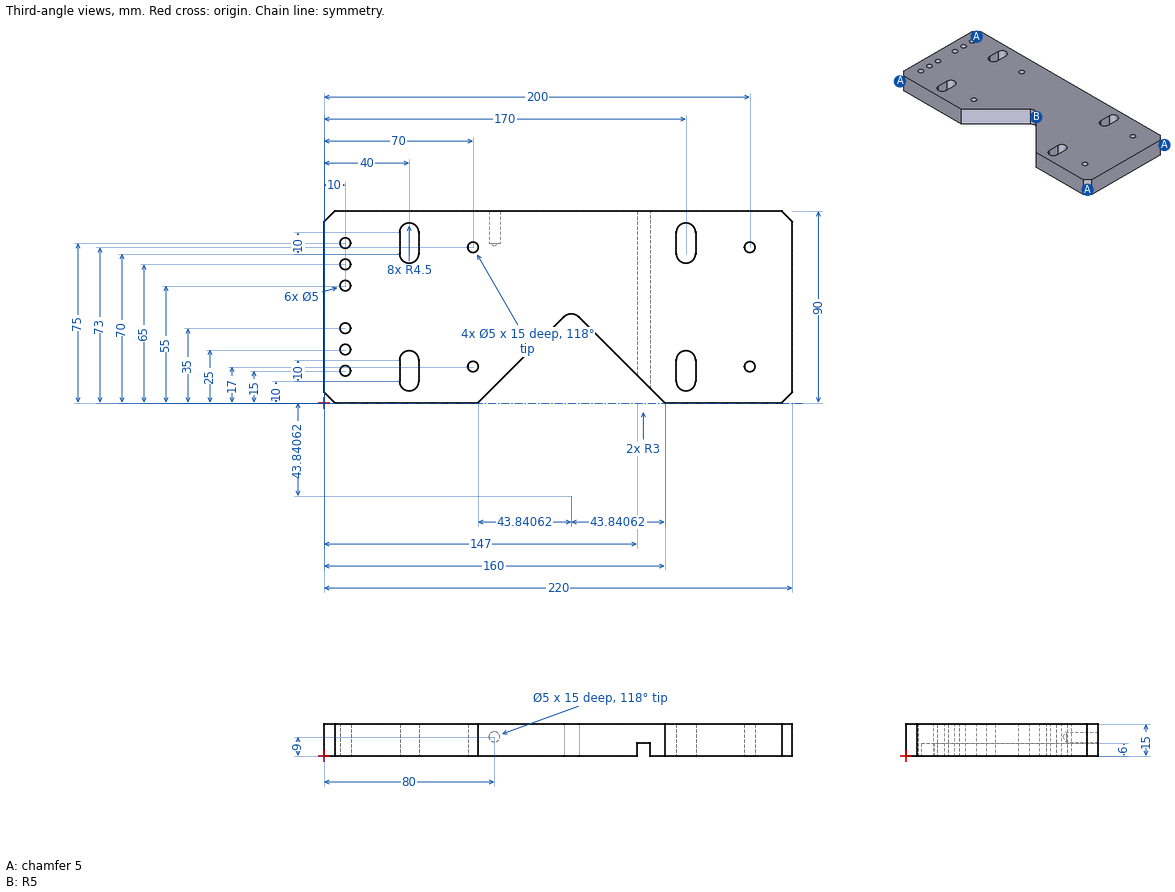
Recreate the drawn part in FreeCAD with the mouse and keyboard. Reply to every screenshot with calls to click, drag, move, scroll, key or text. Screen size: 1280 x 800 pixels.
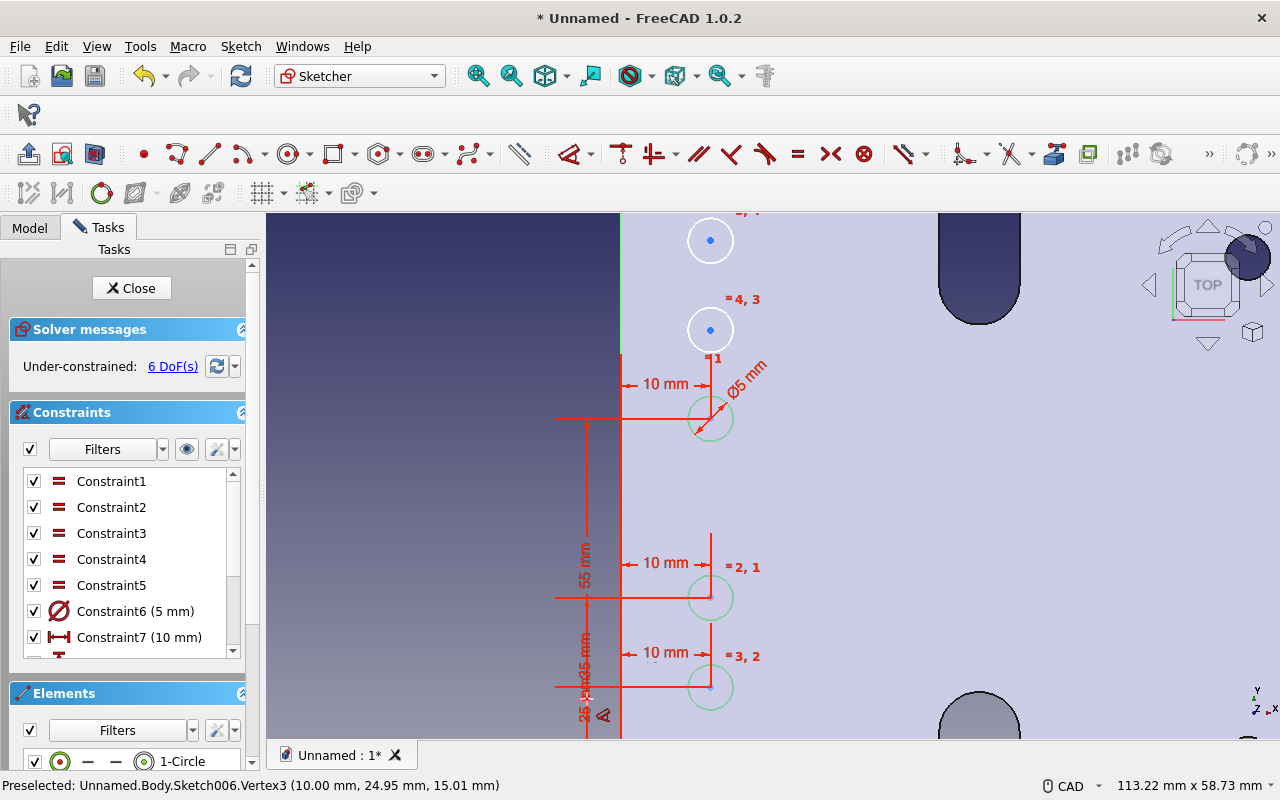
click(711, 330)
click(666, 296)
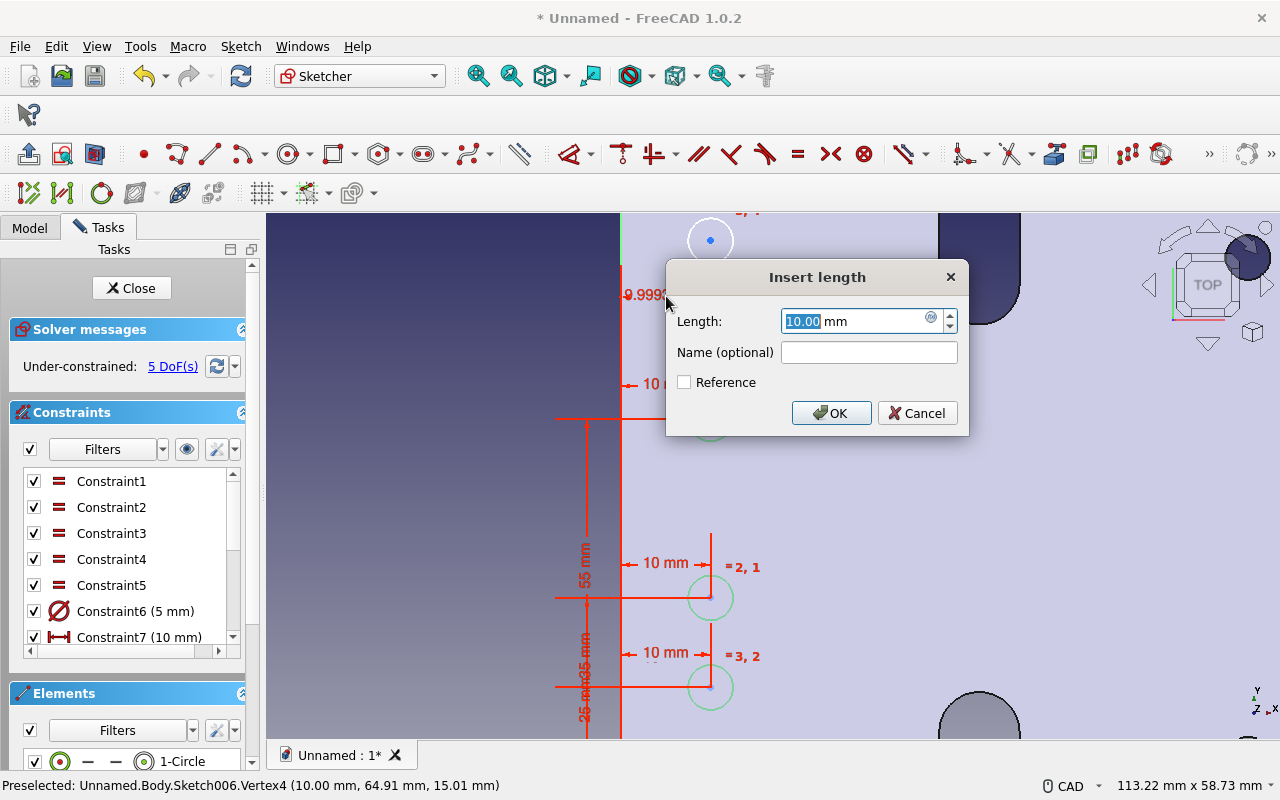
text(10)
key(Return)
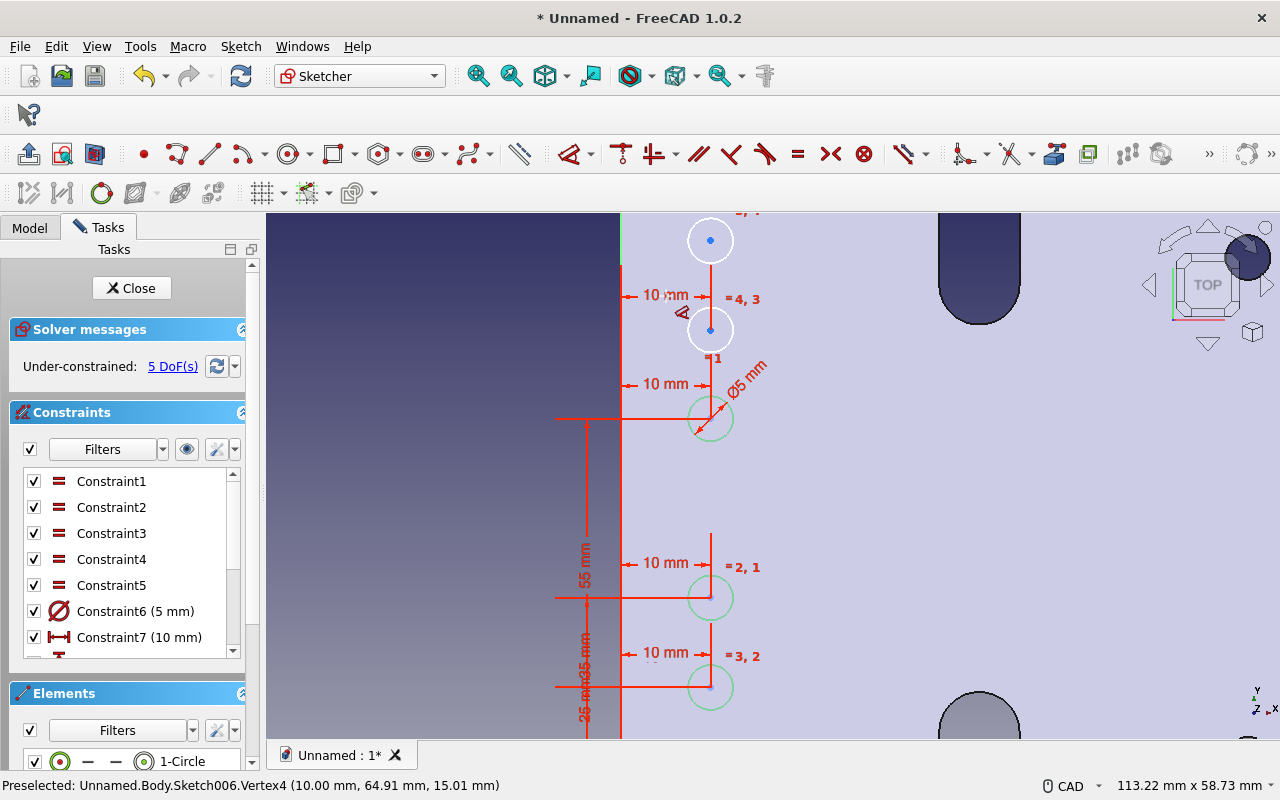
click(711, 330)
click(587, 521)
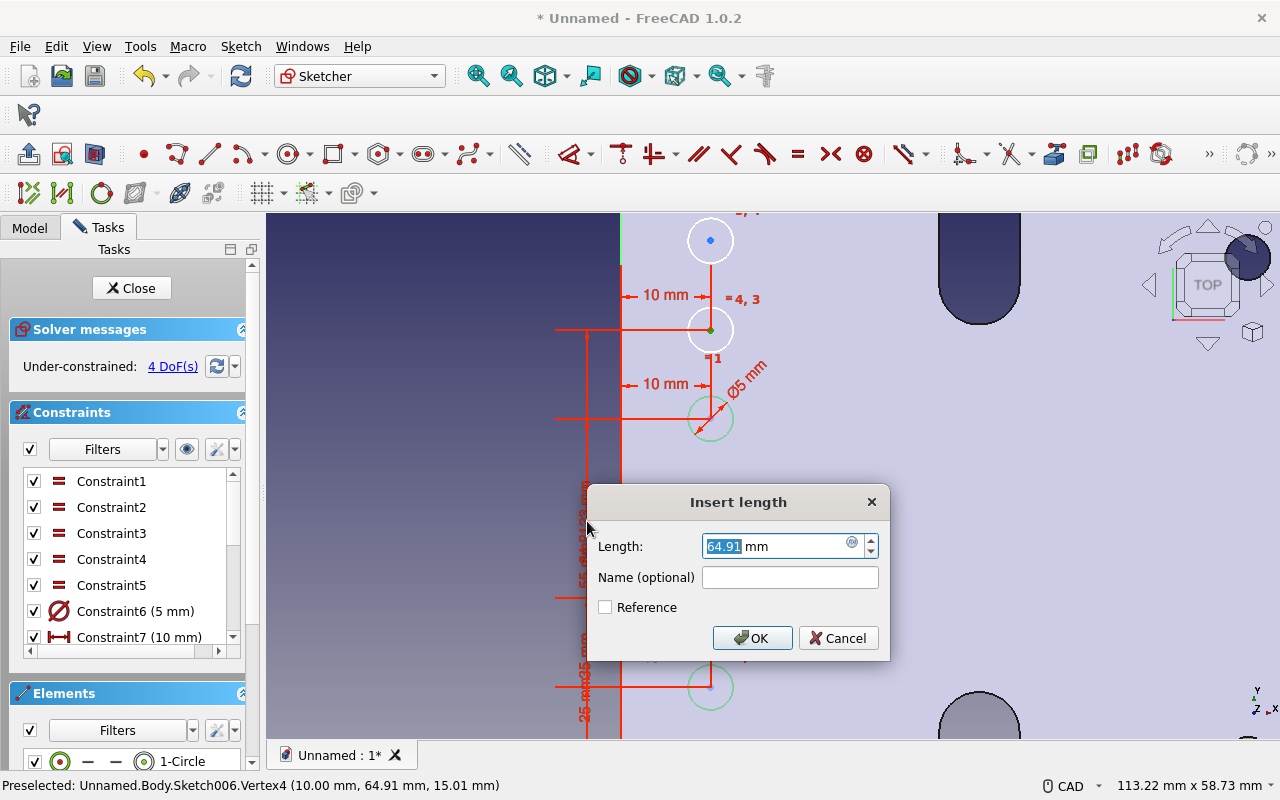
text(65)
key(Return)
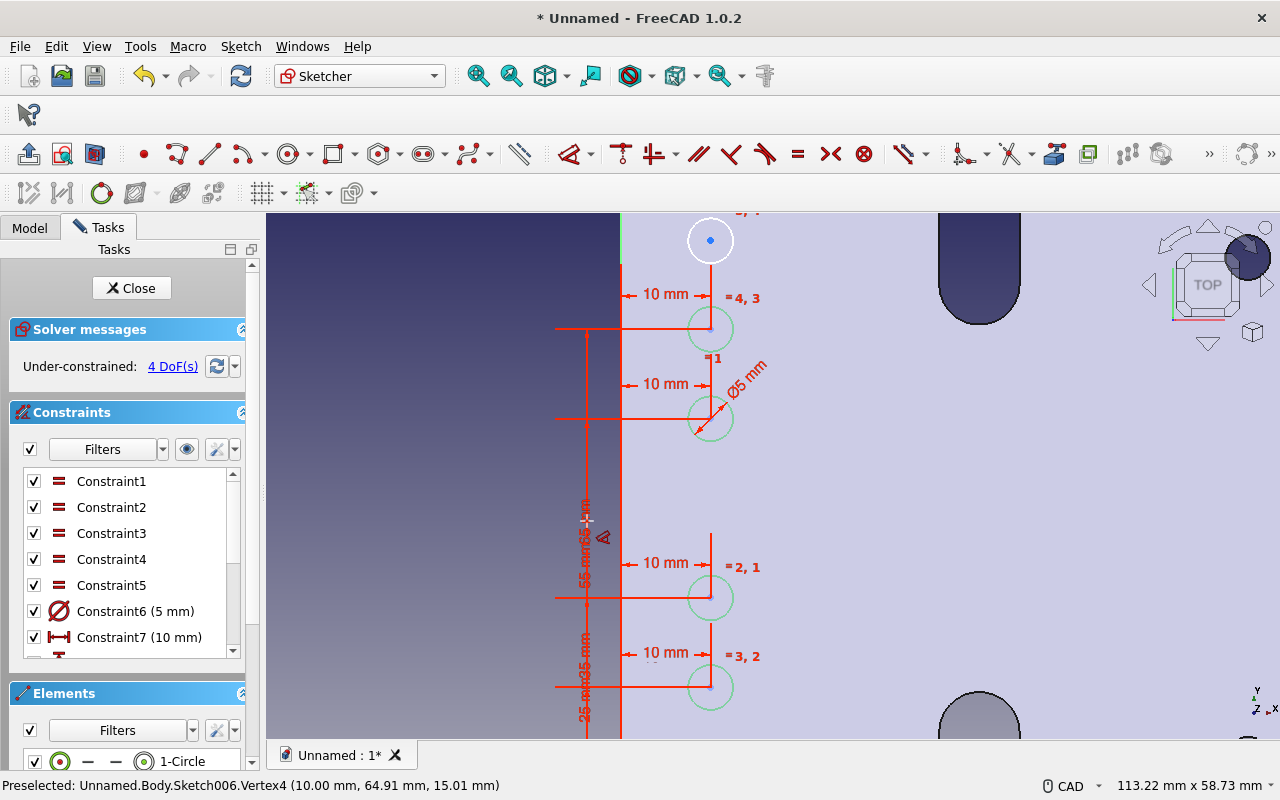
scroll(727, 404, down, 4)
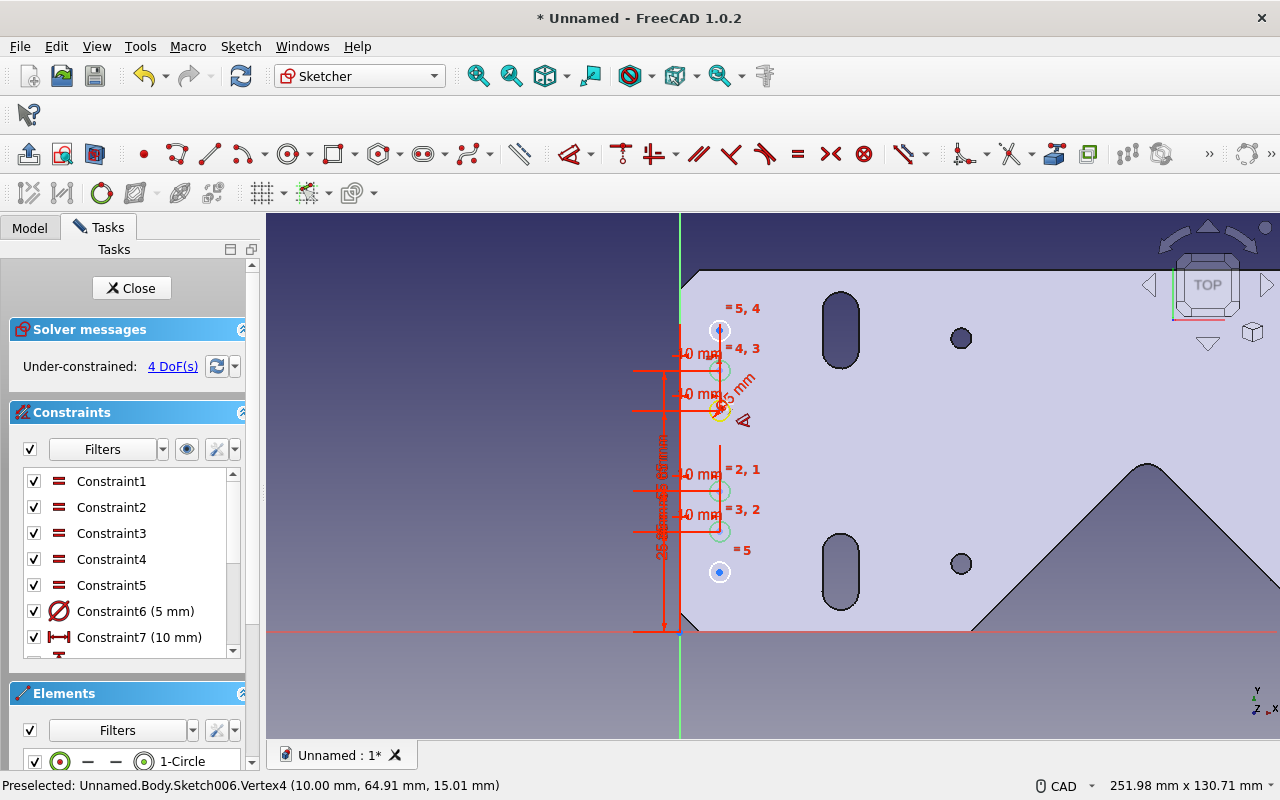
click(720, 331)
click(700, 666)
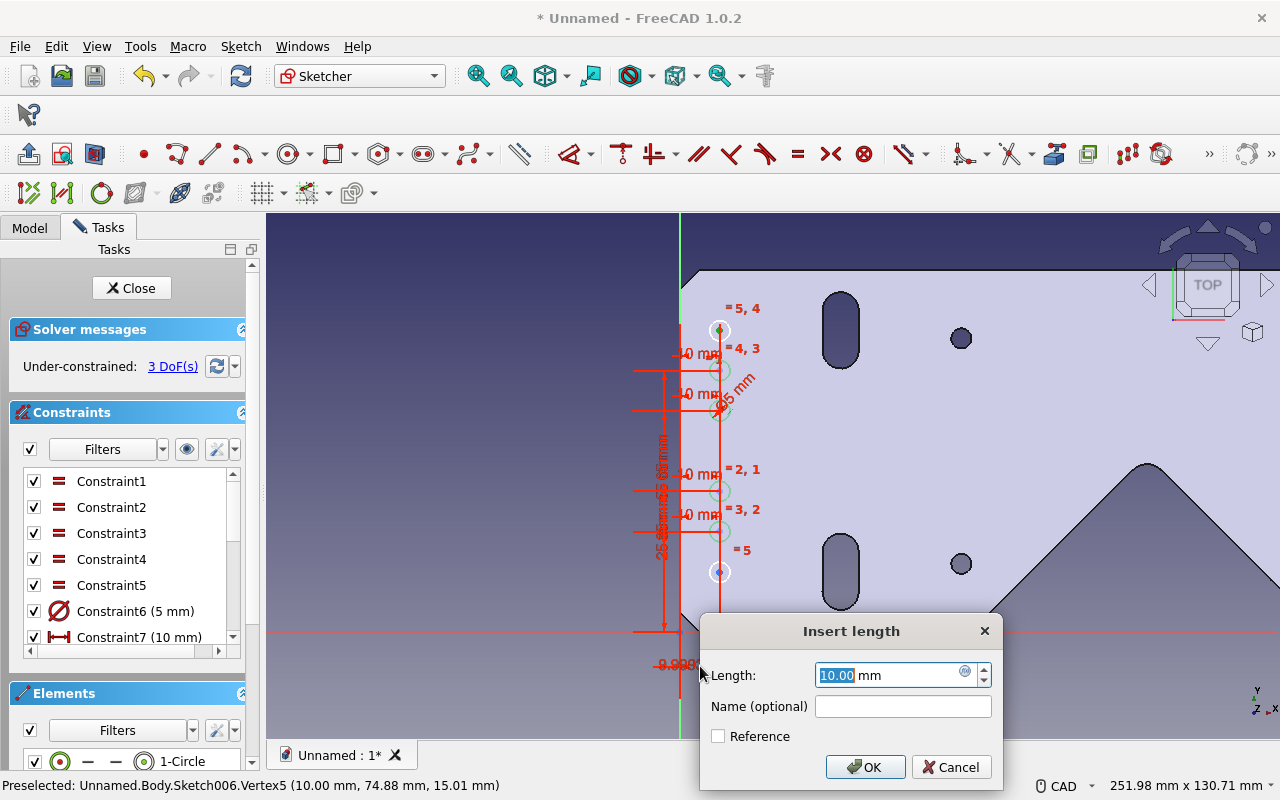
text(10)
key(Return)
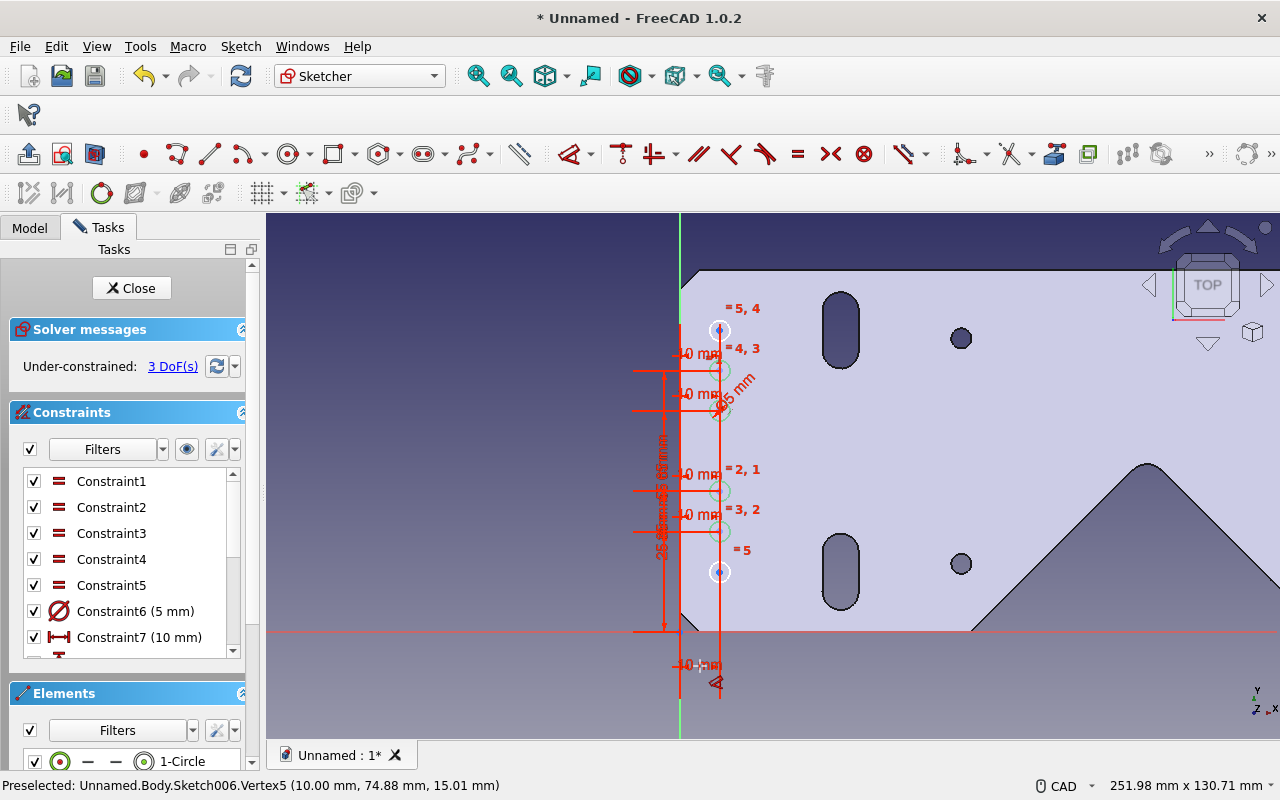
click(720, 331)
click(646, 587)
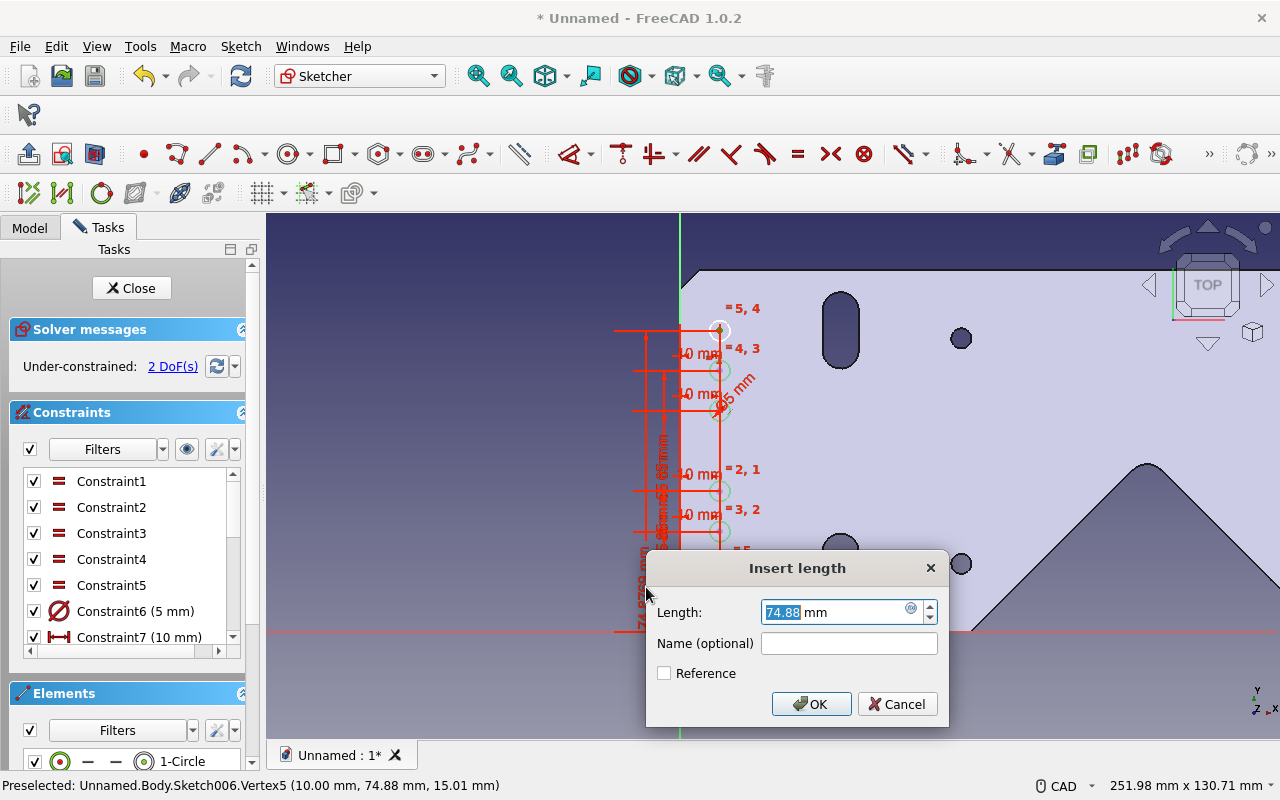
text(75)
key(Return)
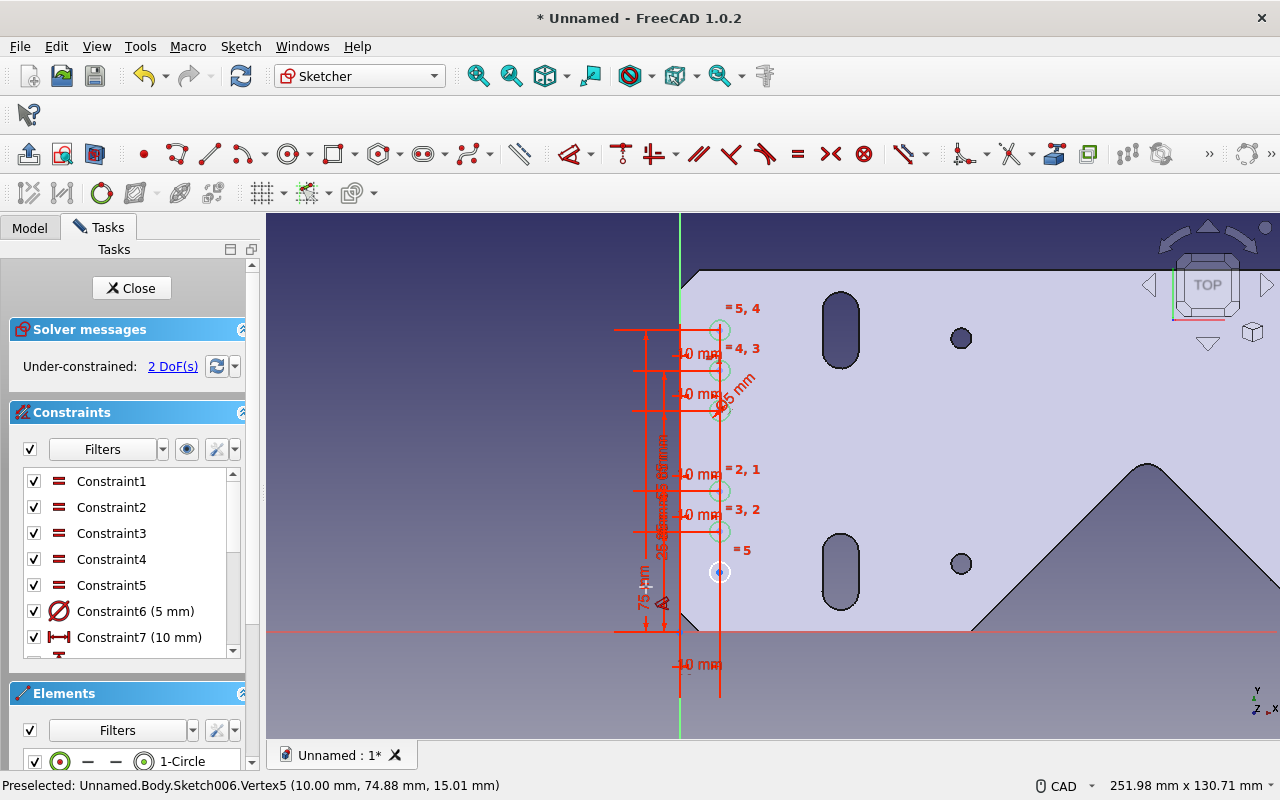
click(720, 572)
click(700, 690)